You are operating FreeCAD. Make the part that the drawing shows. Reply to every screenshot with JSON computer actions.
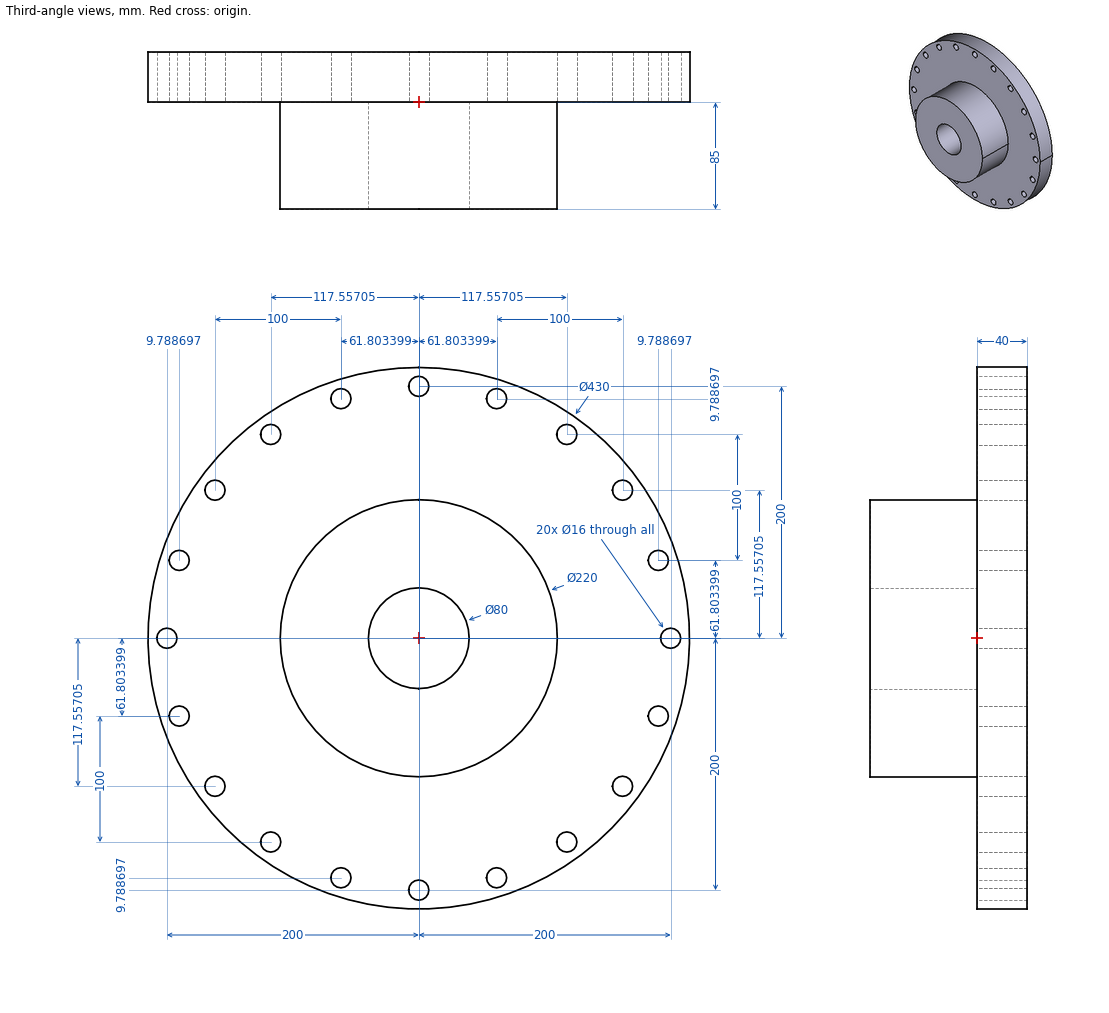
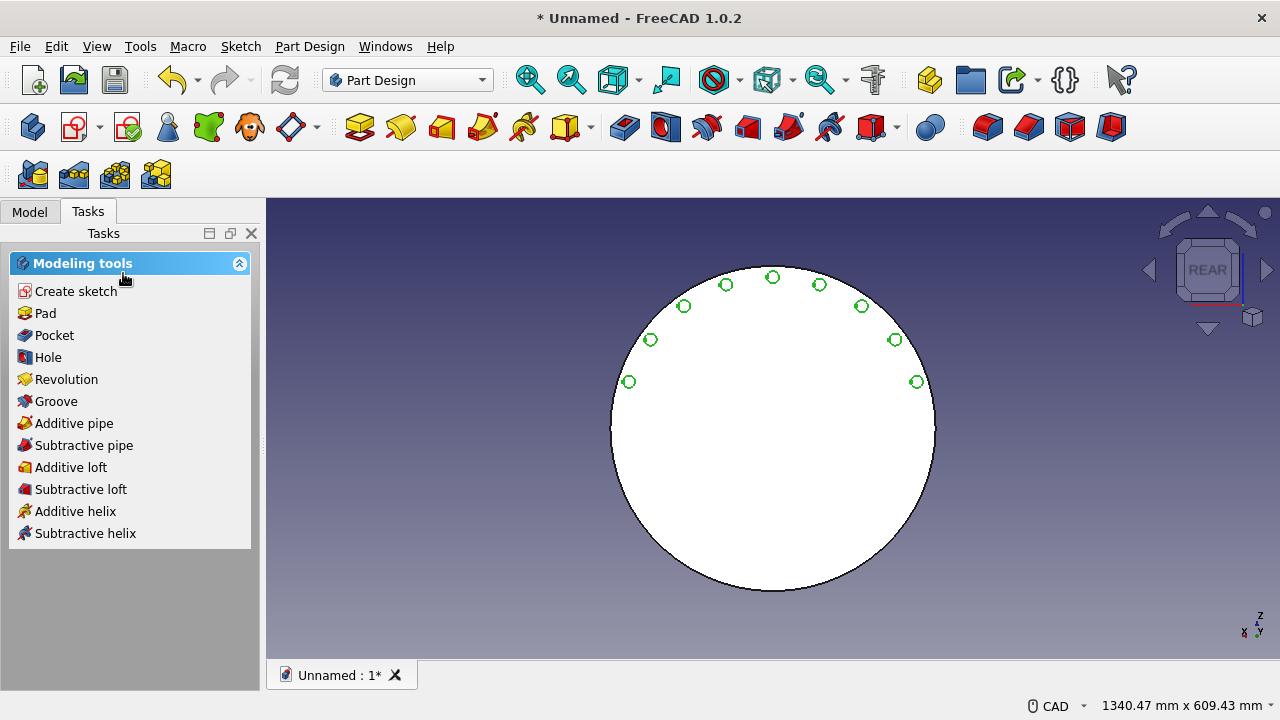
{"action": "left_click", "coordinate": [666, 128]}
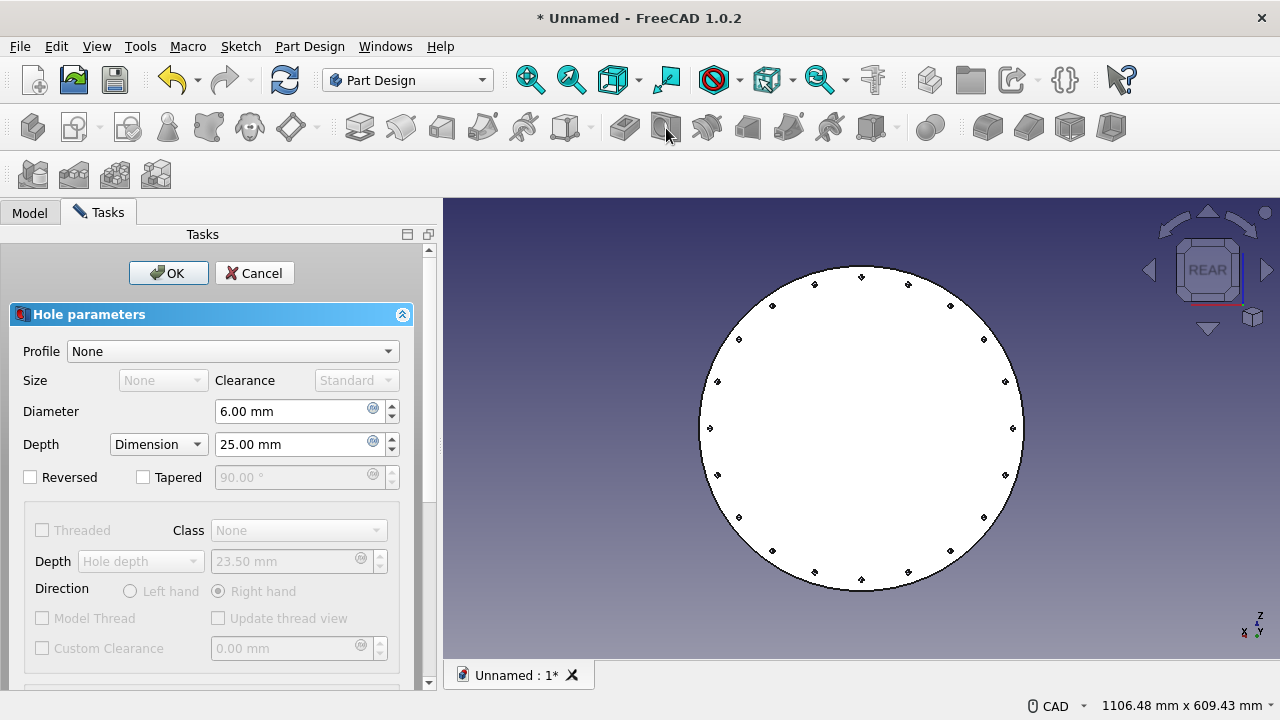
{"action": "triple_click", "coordinate": [300, 412]}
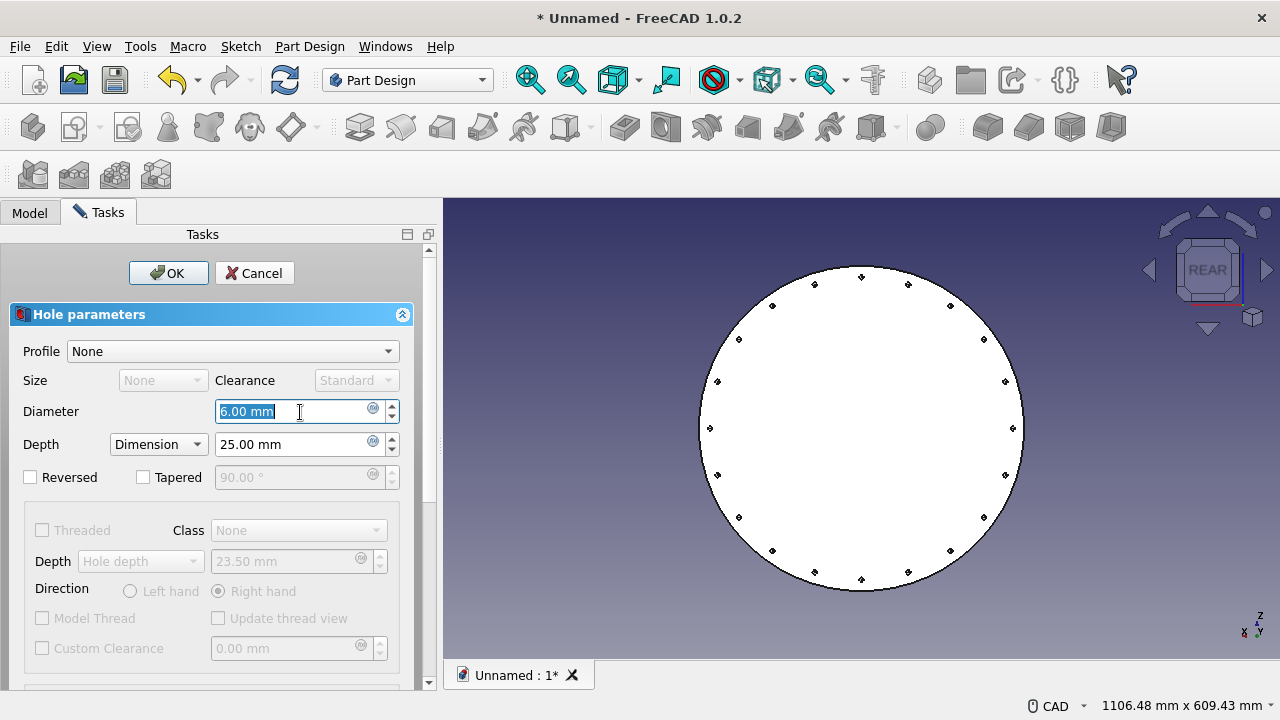
{"action": "type", "text": "16"}
{"action": "key", "text": "Tab"}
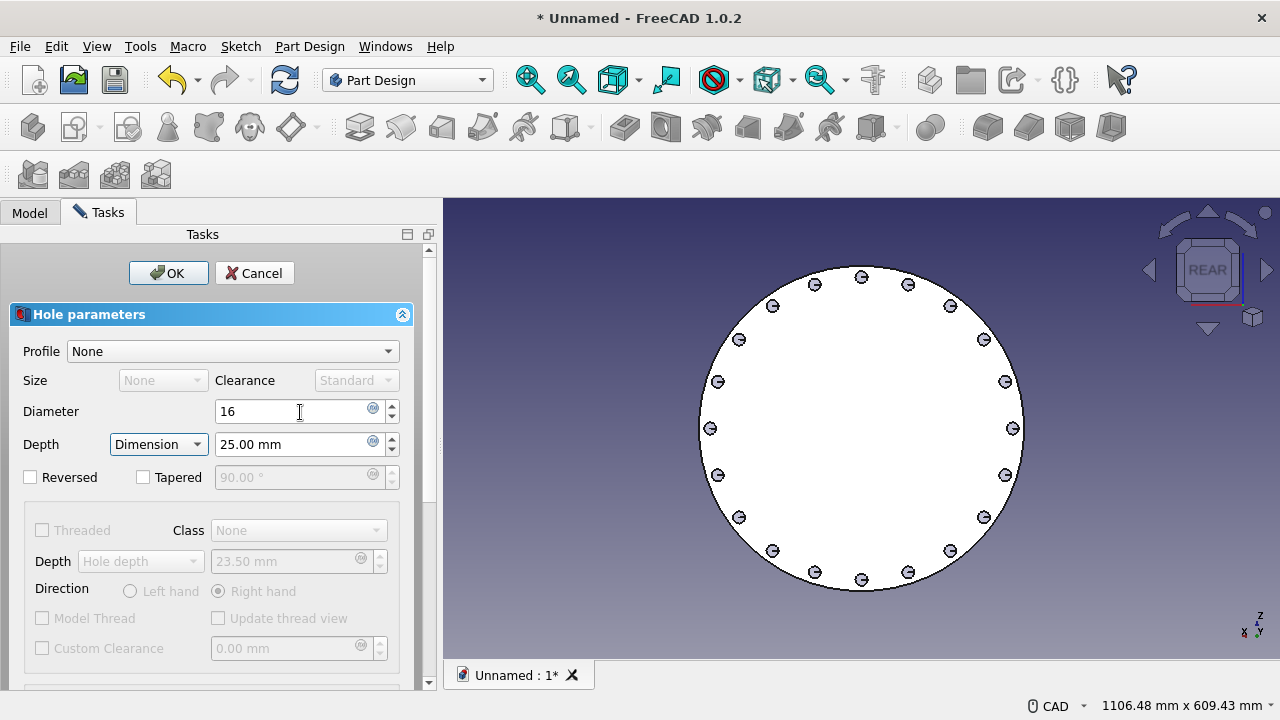
{"action": "left_click", "coordinate": [160, 444]}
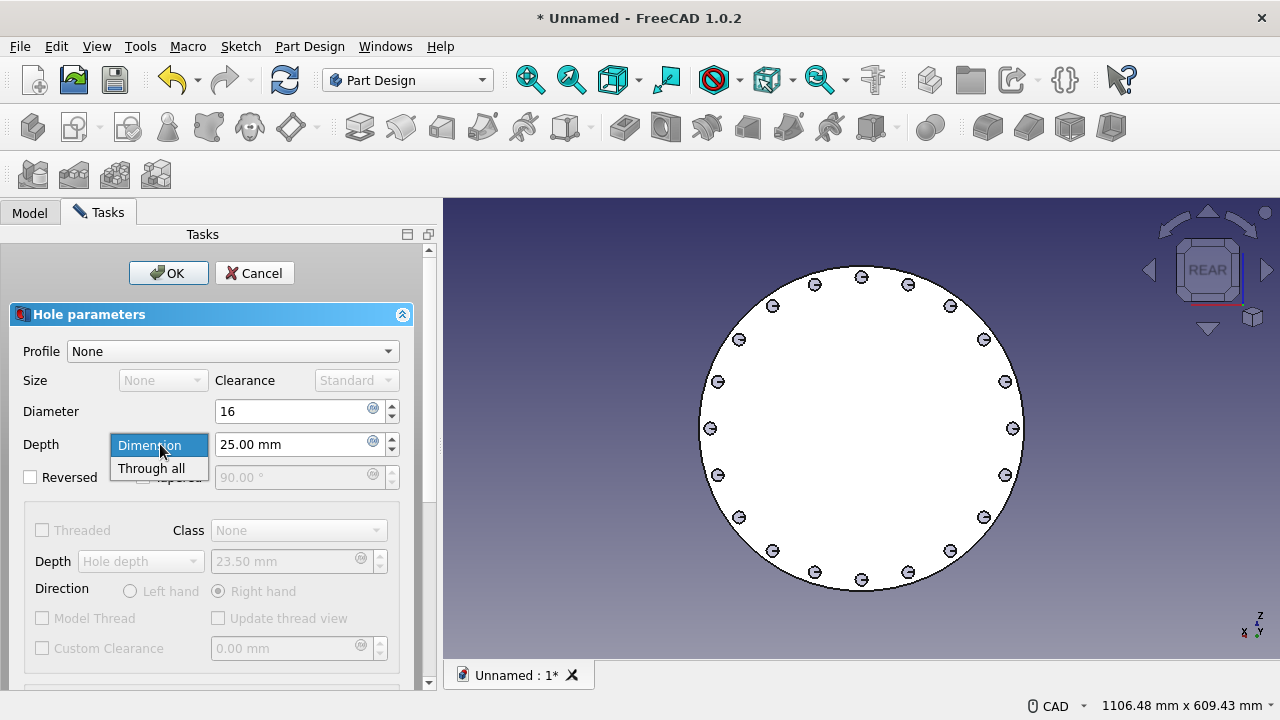
{"action": "left_click", "coordinate": [158, 468]}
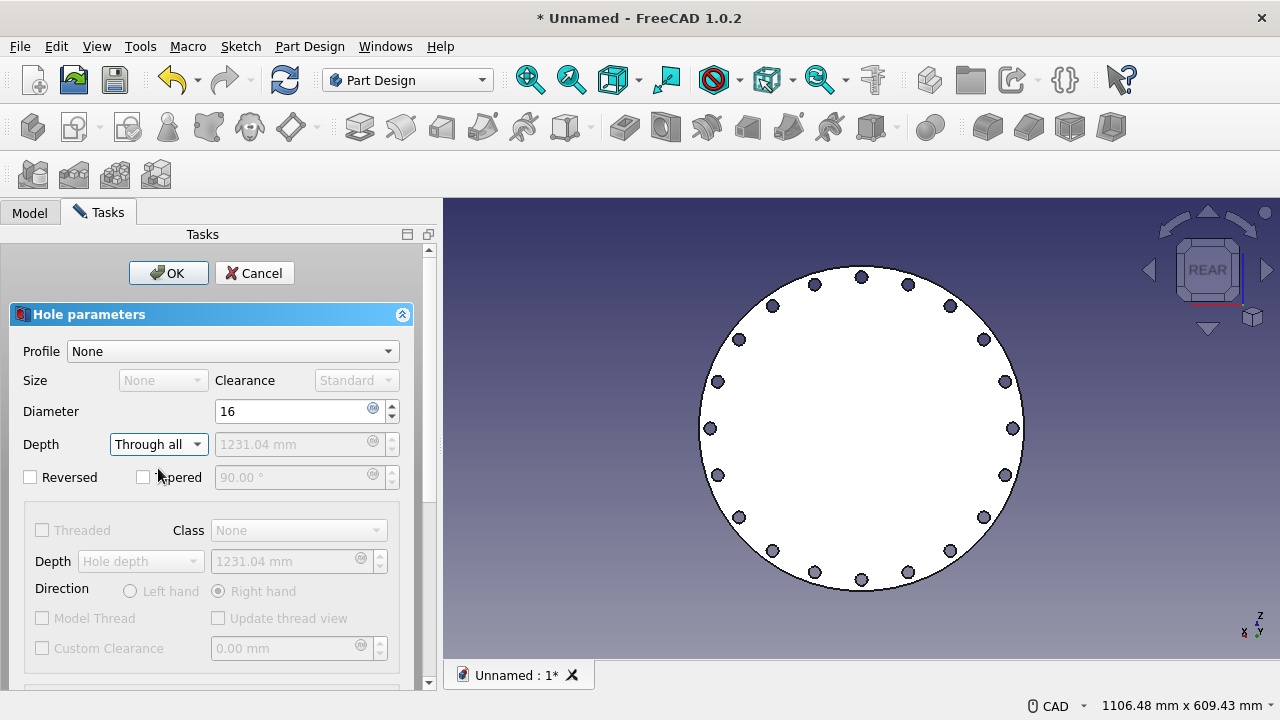
{"action": "left_click", "coordinate": [169, 273]}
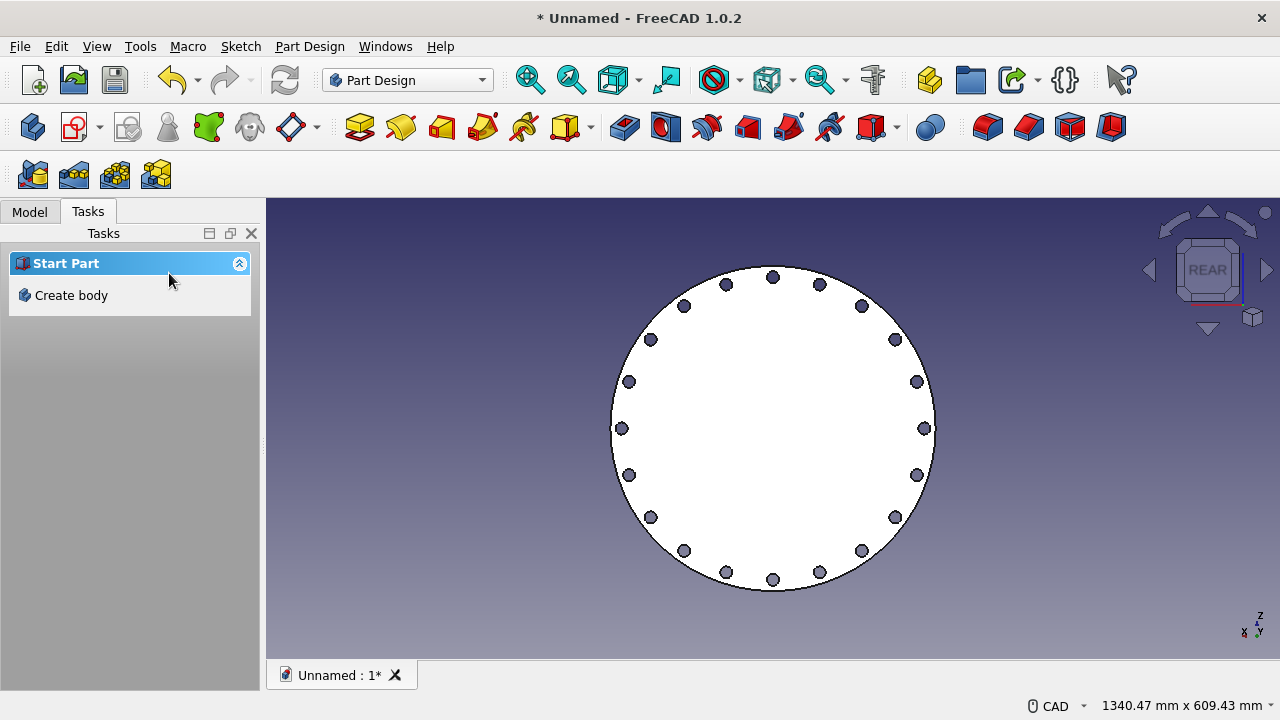
{"action": "key", "text": "0"}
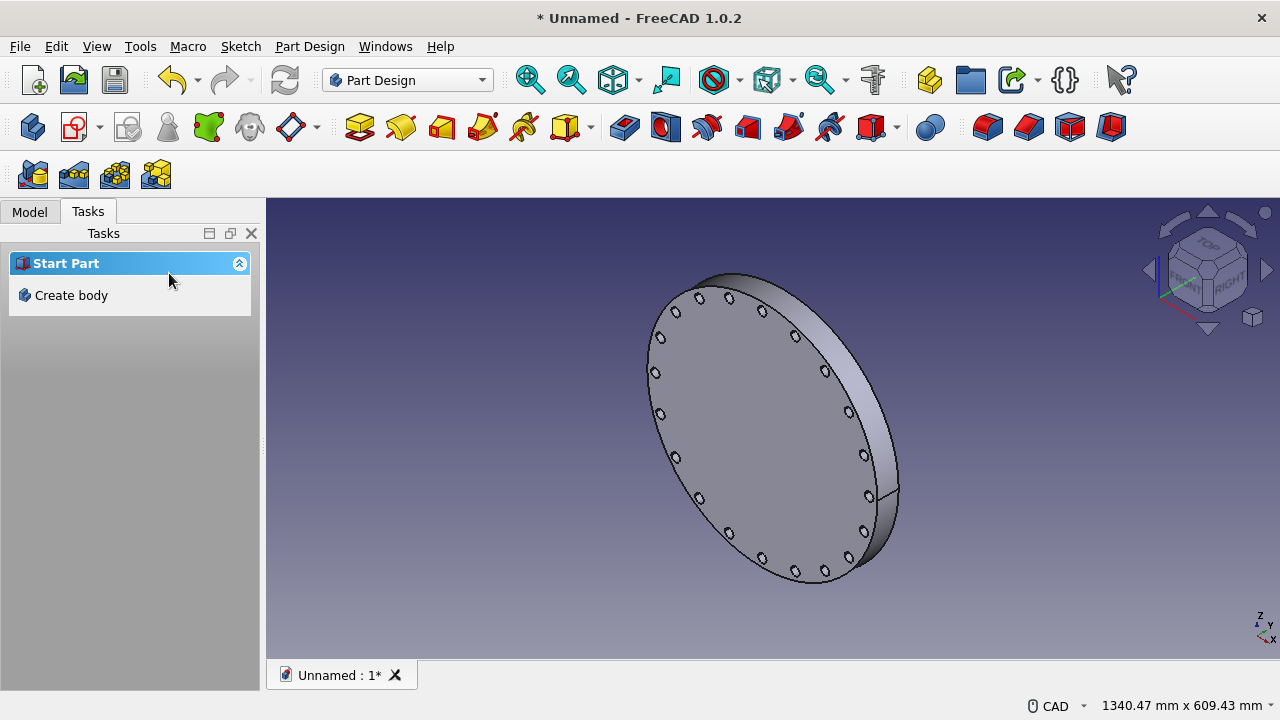
{"action": "left_click", "coordinate": [762, 434]}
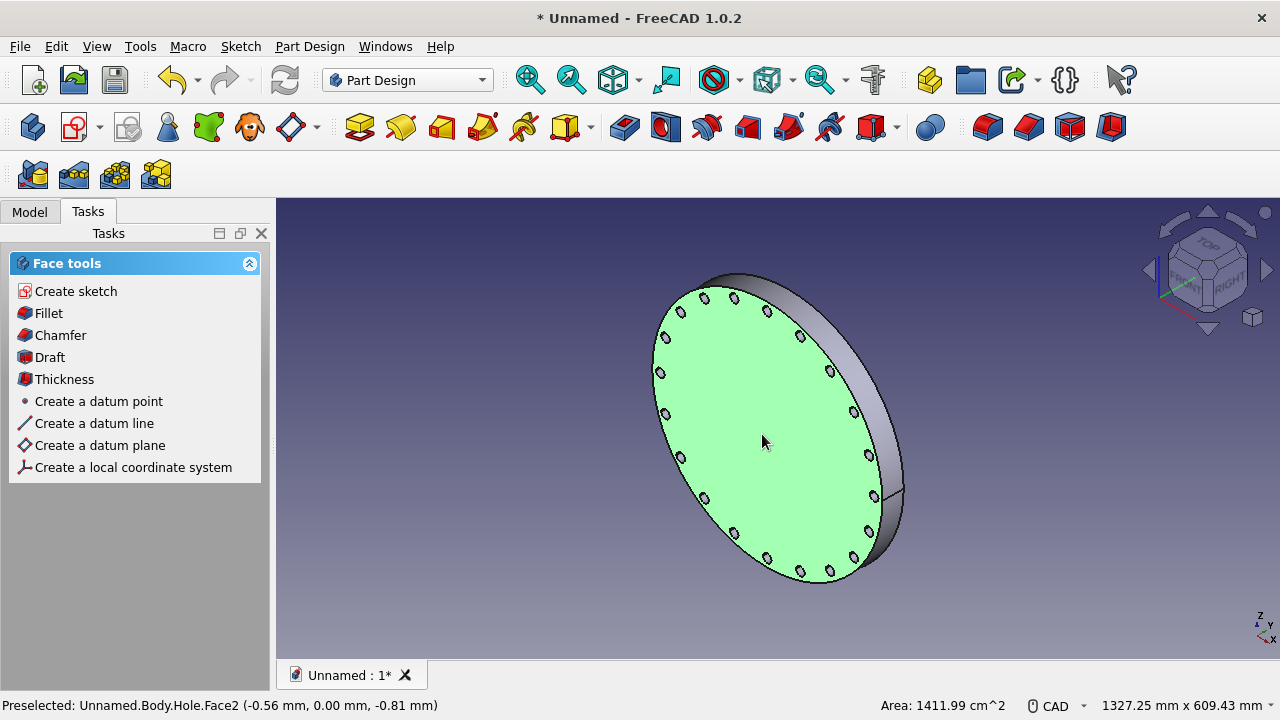
{"action": "left_click", "coordinate": [74, 128]}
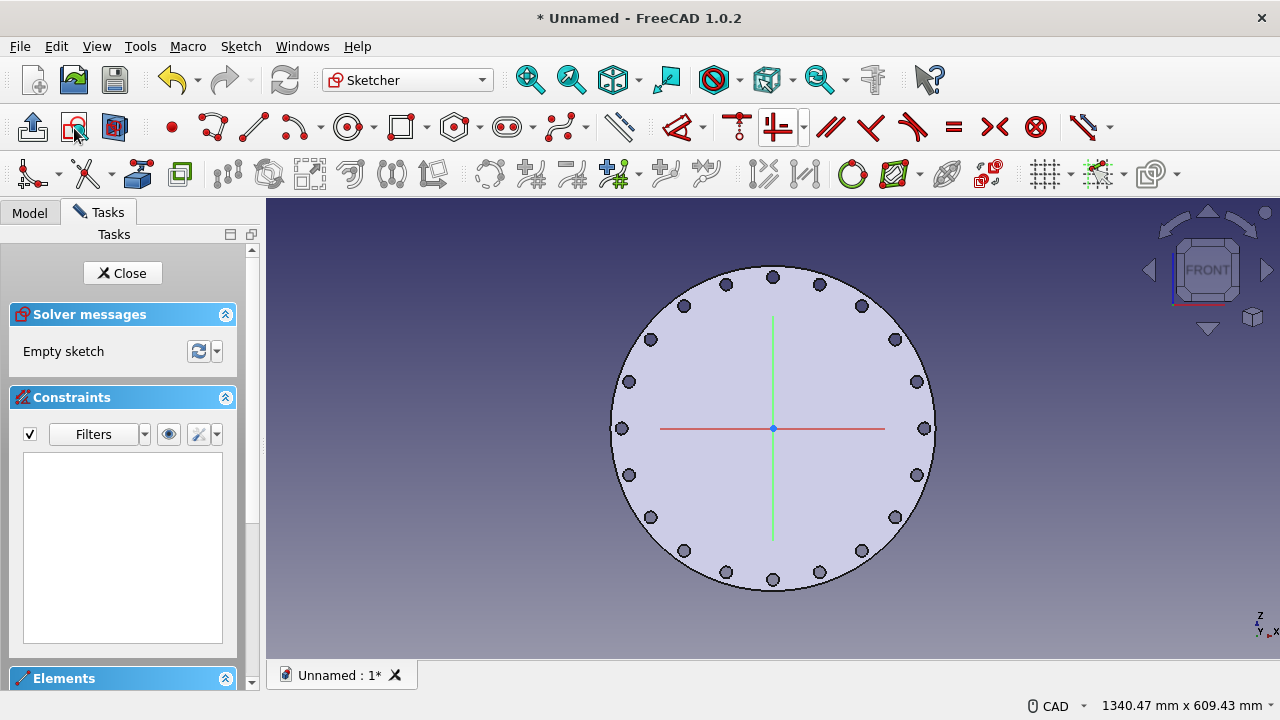
{"action": "scroll", "coordinate": [856, 429], "scroll_direction": "up", "scroll_amount": 3}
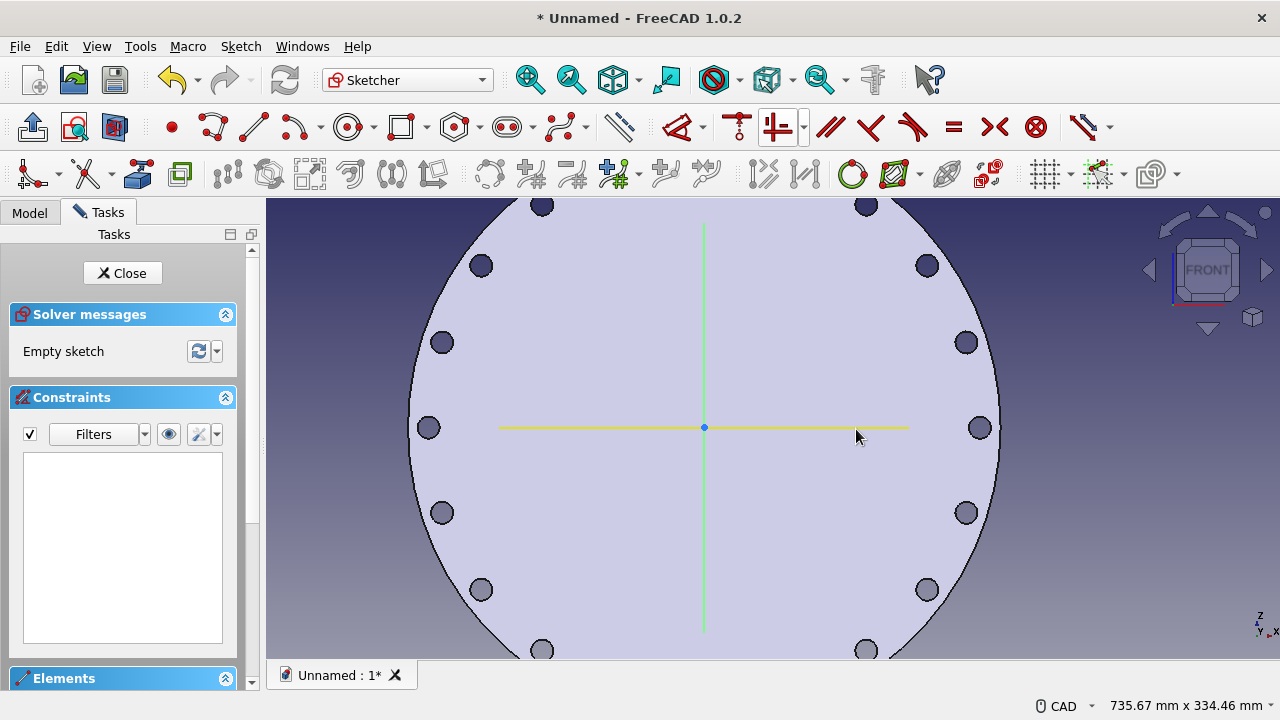
{"action": "key", "text": "g c"}